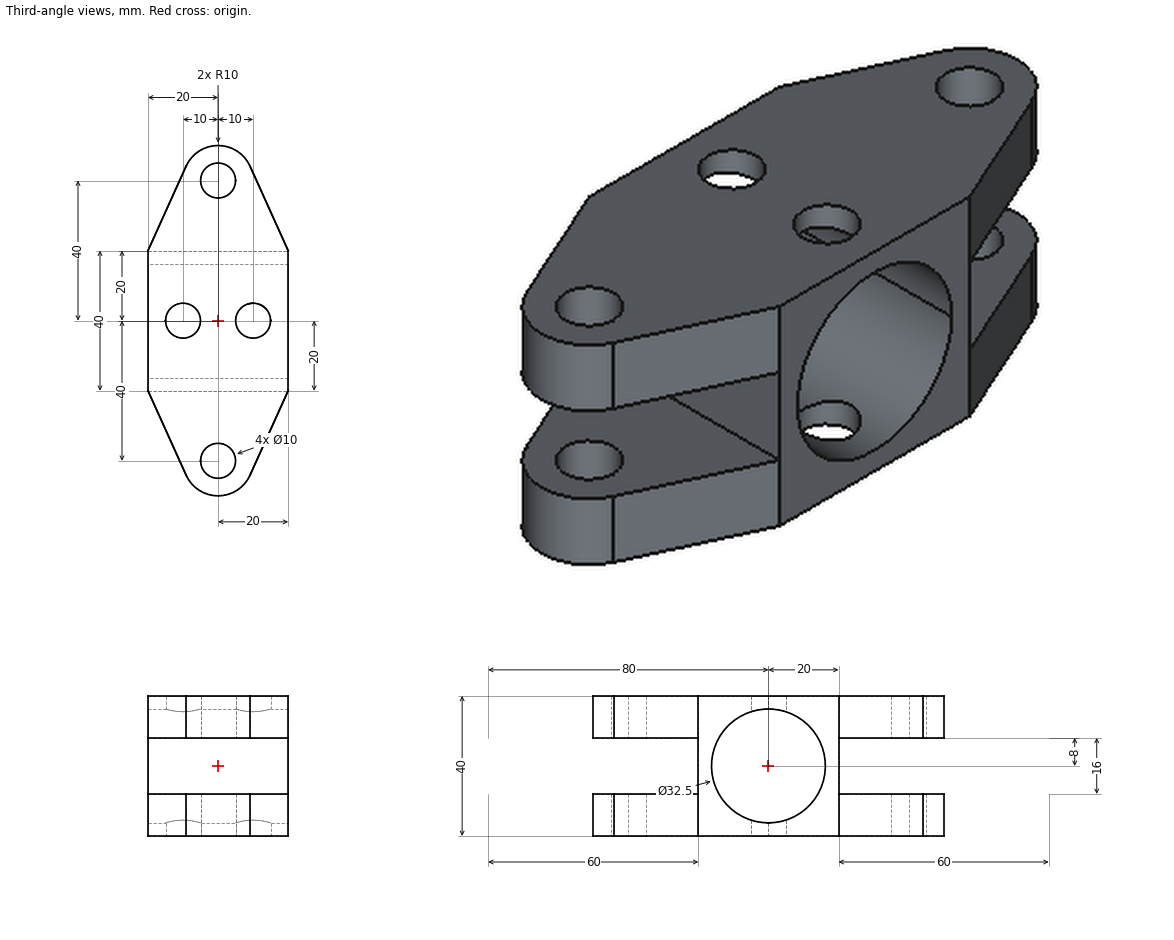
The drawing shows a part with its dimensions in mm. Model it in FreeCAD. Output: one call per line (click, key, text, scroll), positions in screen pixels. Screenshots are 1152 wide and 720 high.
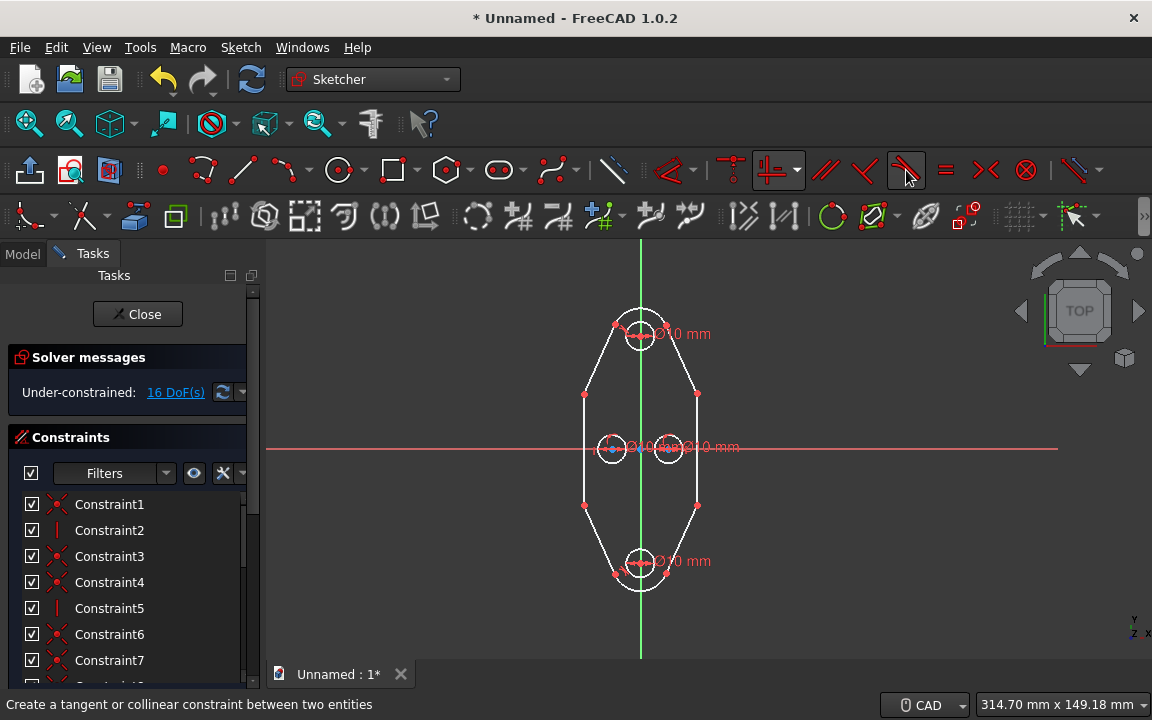
click(675, 554)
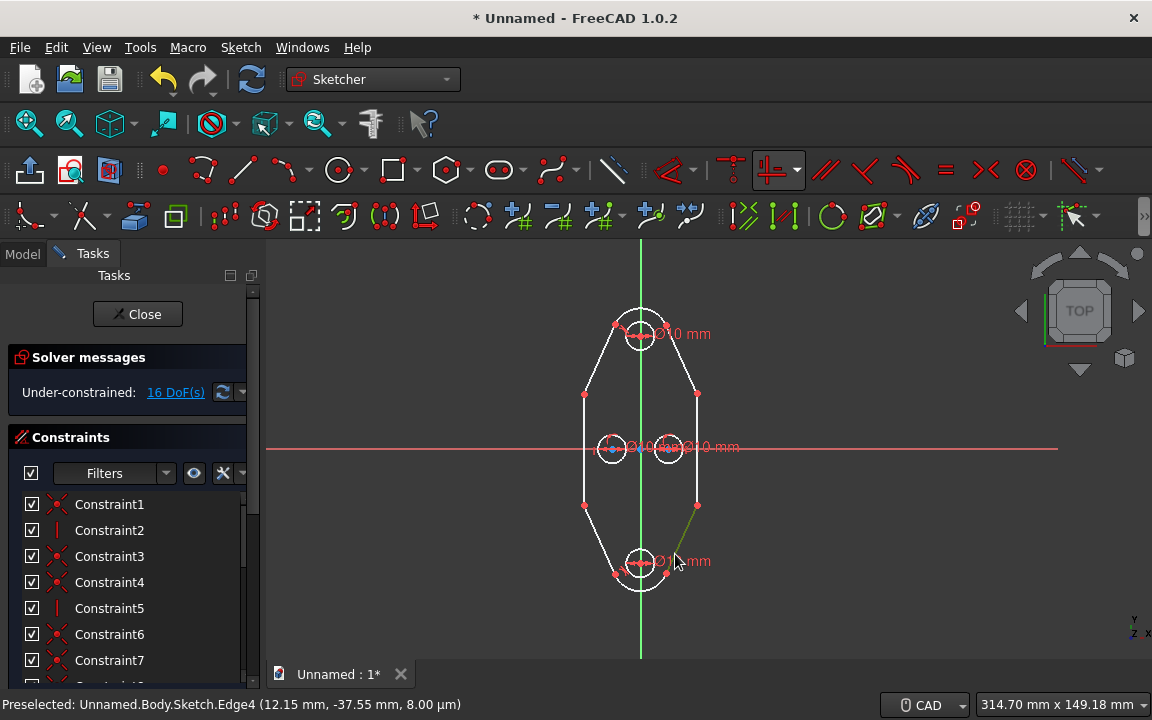
click(628, 588)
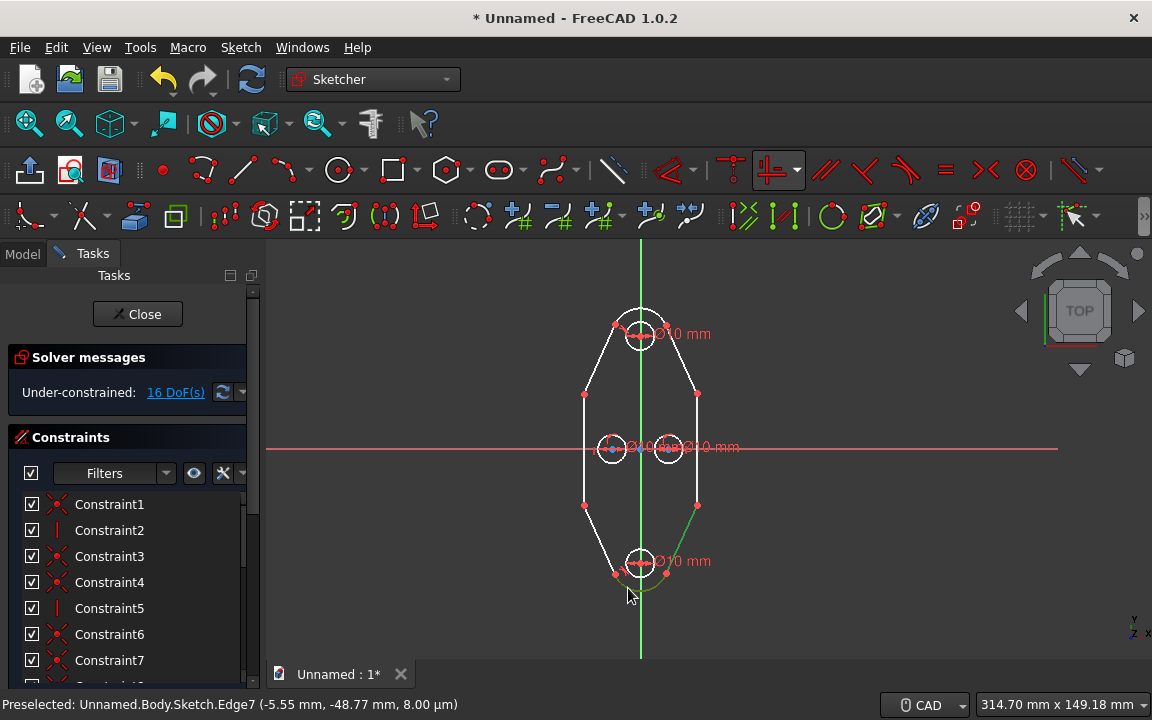
click(906, 170)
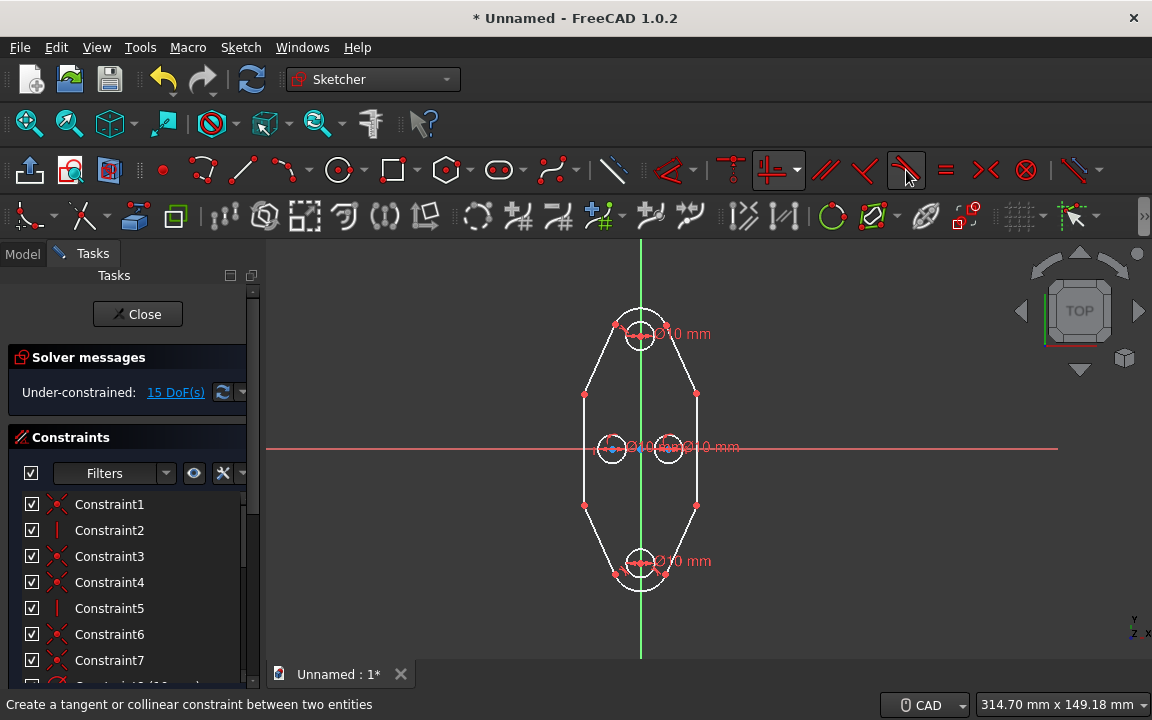
click(688, 374)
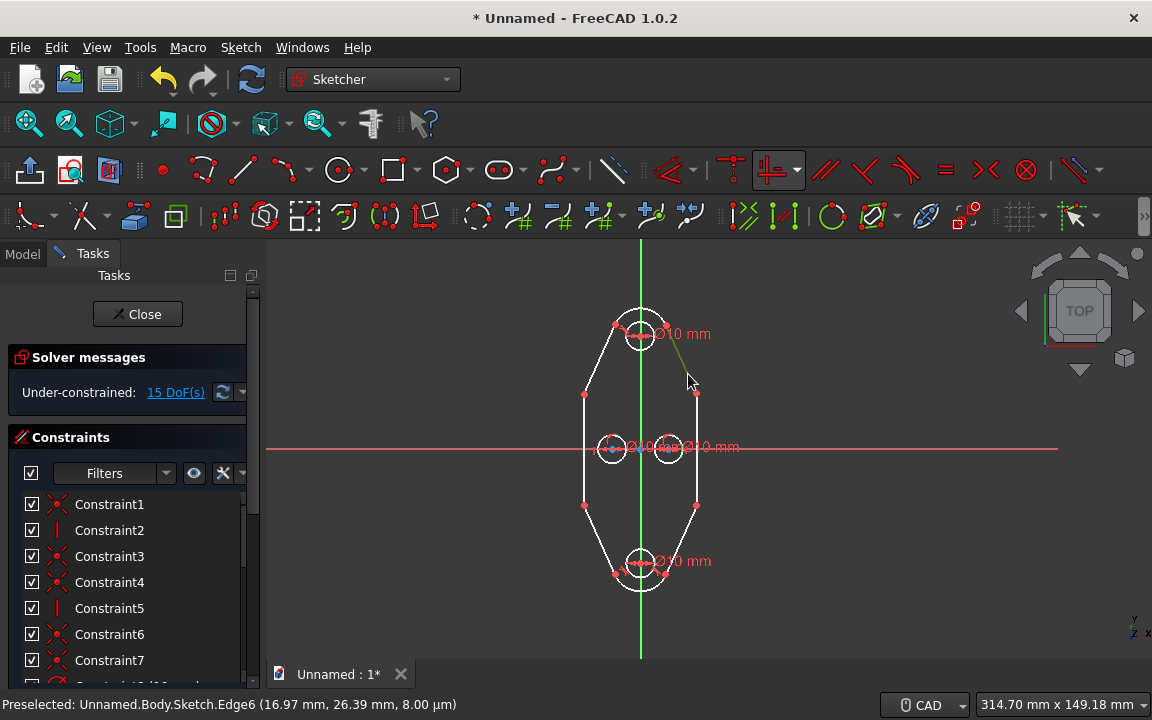
click(653, 312)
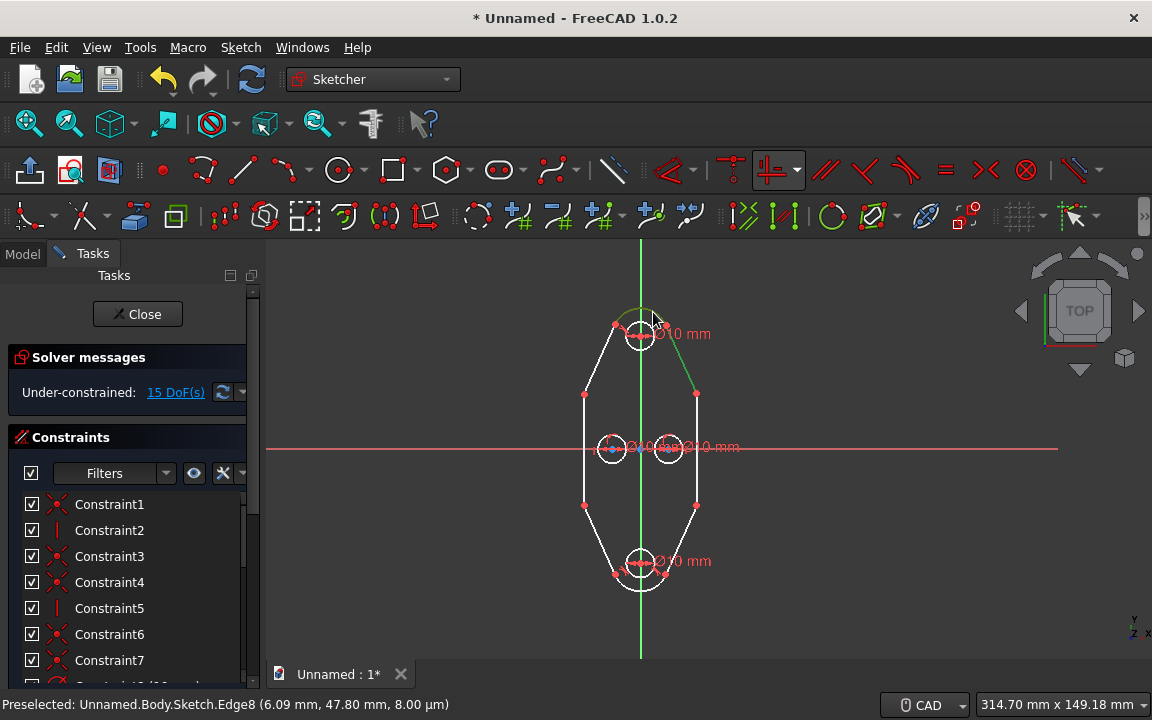
click(906, 170)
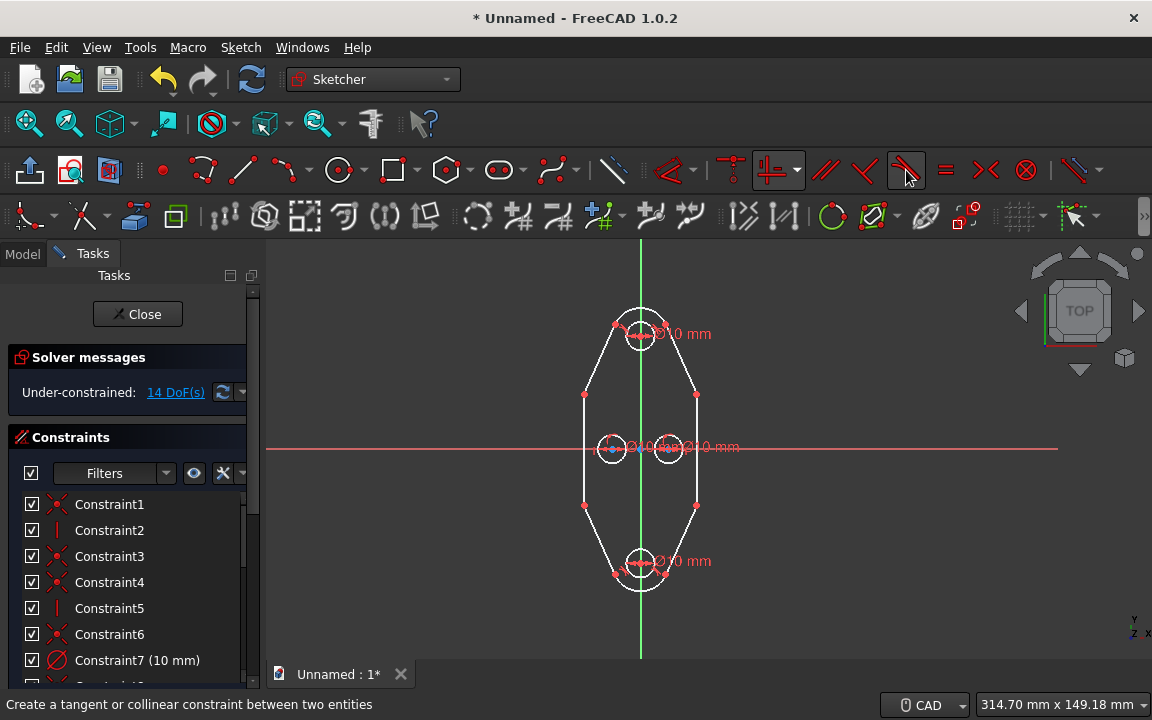
click(628, 588)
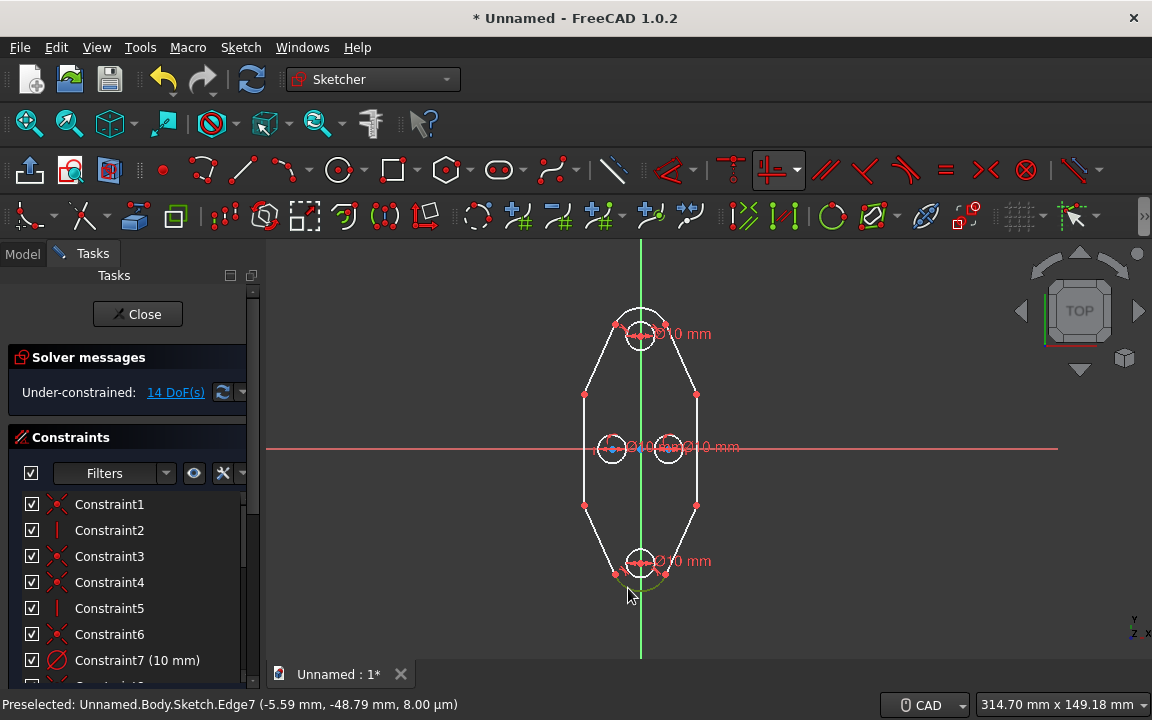
click(653, 311)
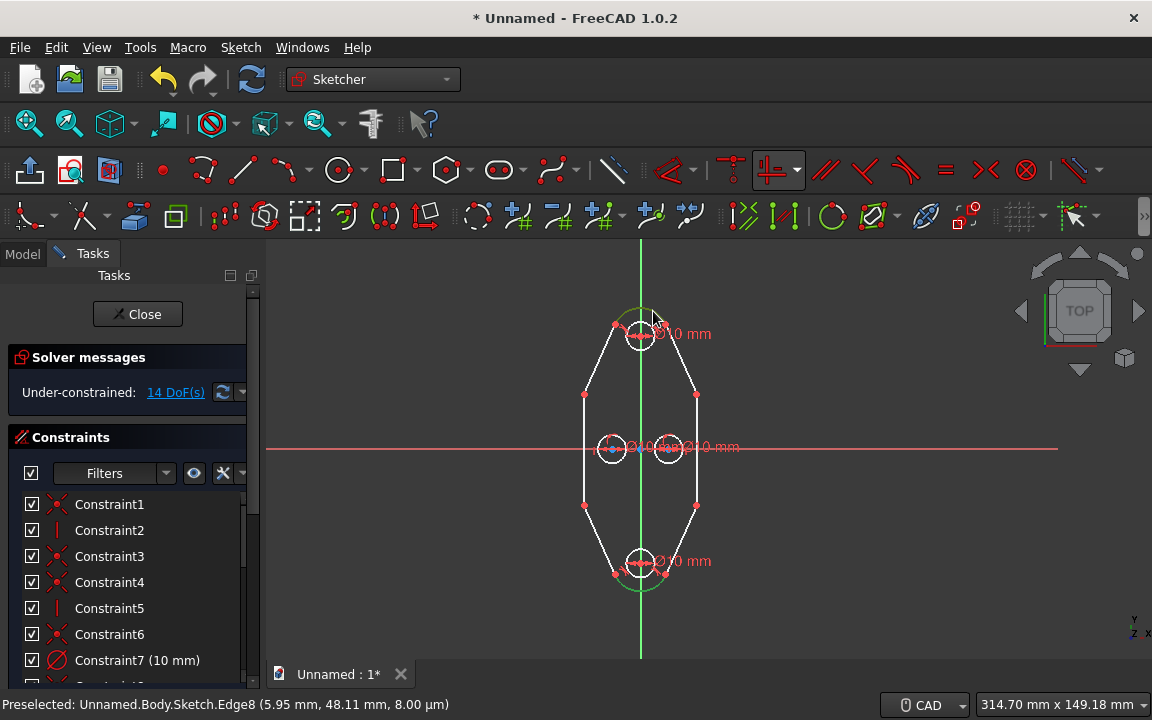
click(946, 170)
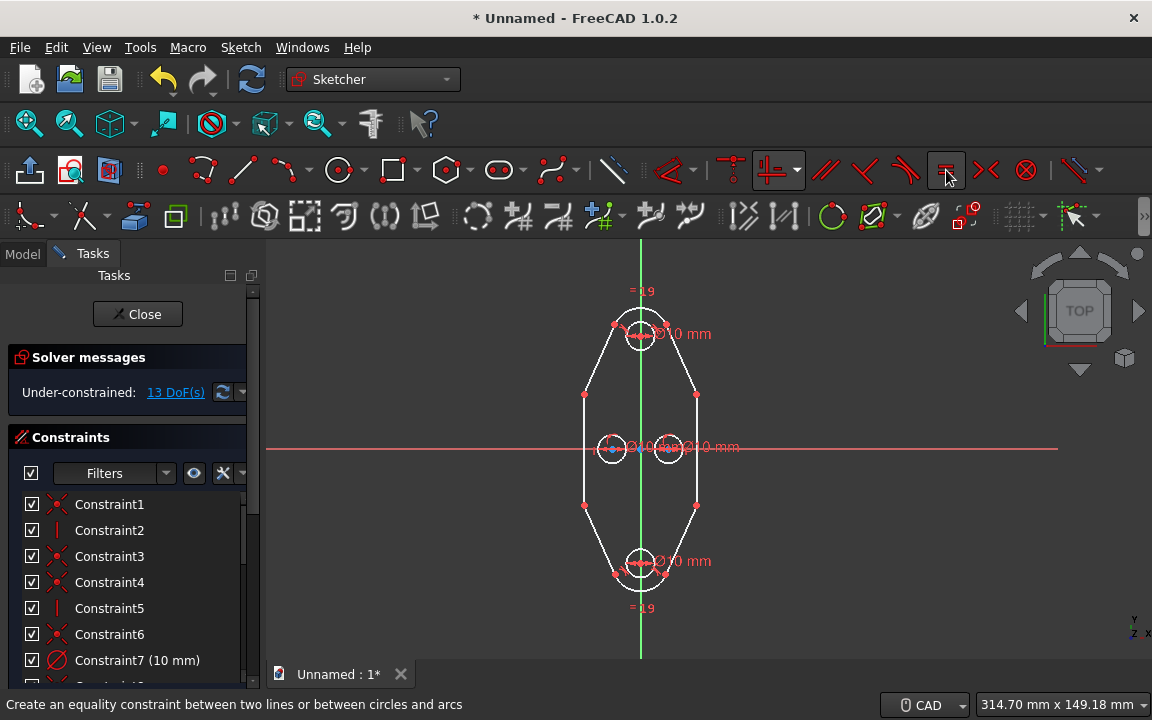
click(640, 563)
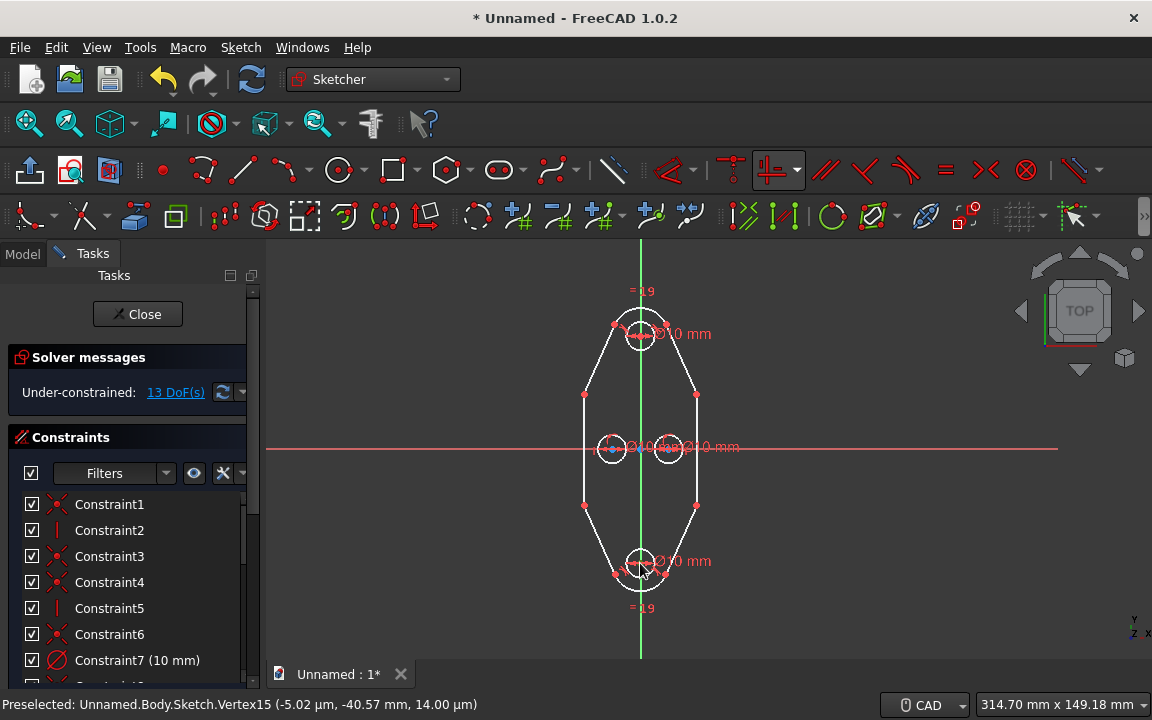
click(641, 501)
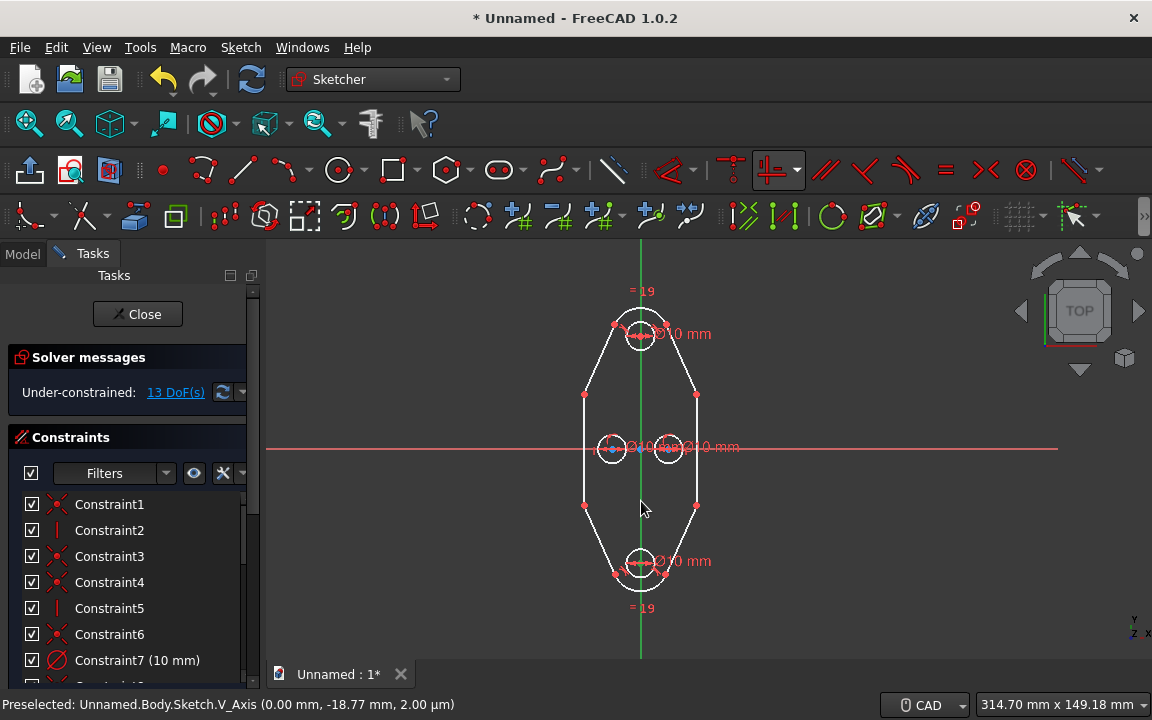
click(732, 170)